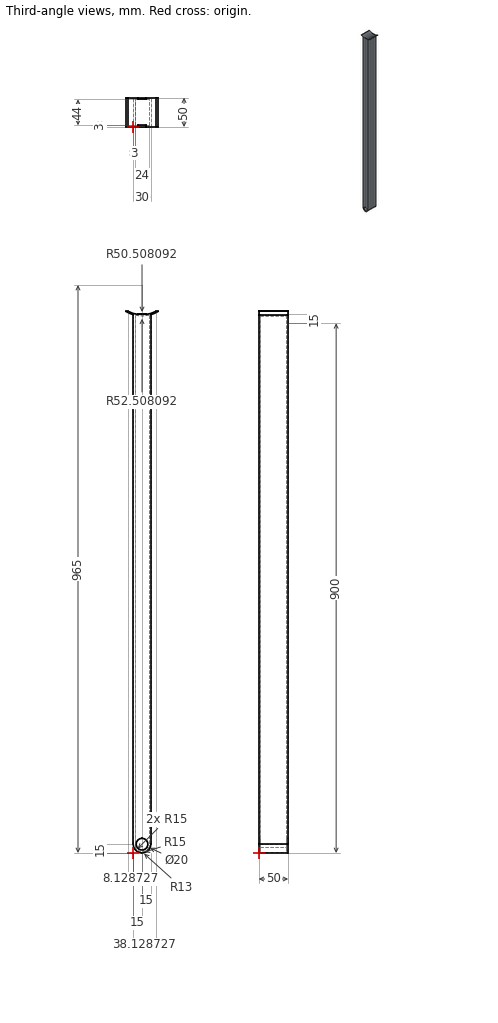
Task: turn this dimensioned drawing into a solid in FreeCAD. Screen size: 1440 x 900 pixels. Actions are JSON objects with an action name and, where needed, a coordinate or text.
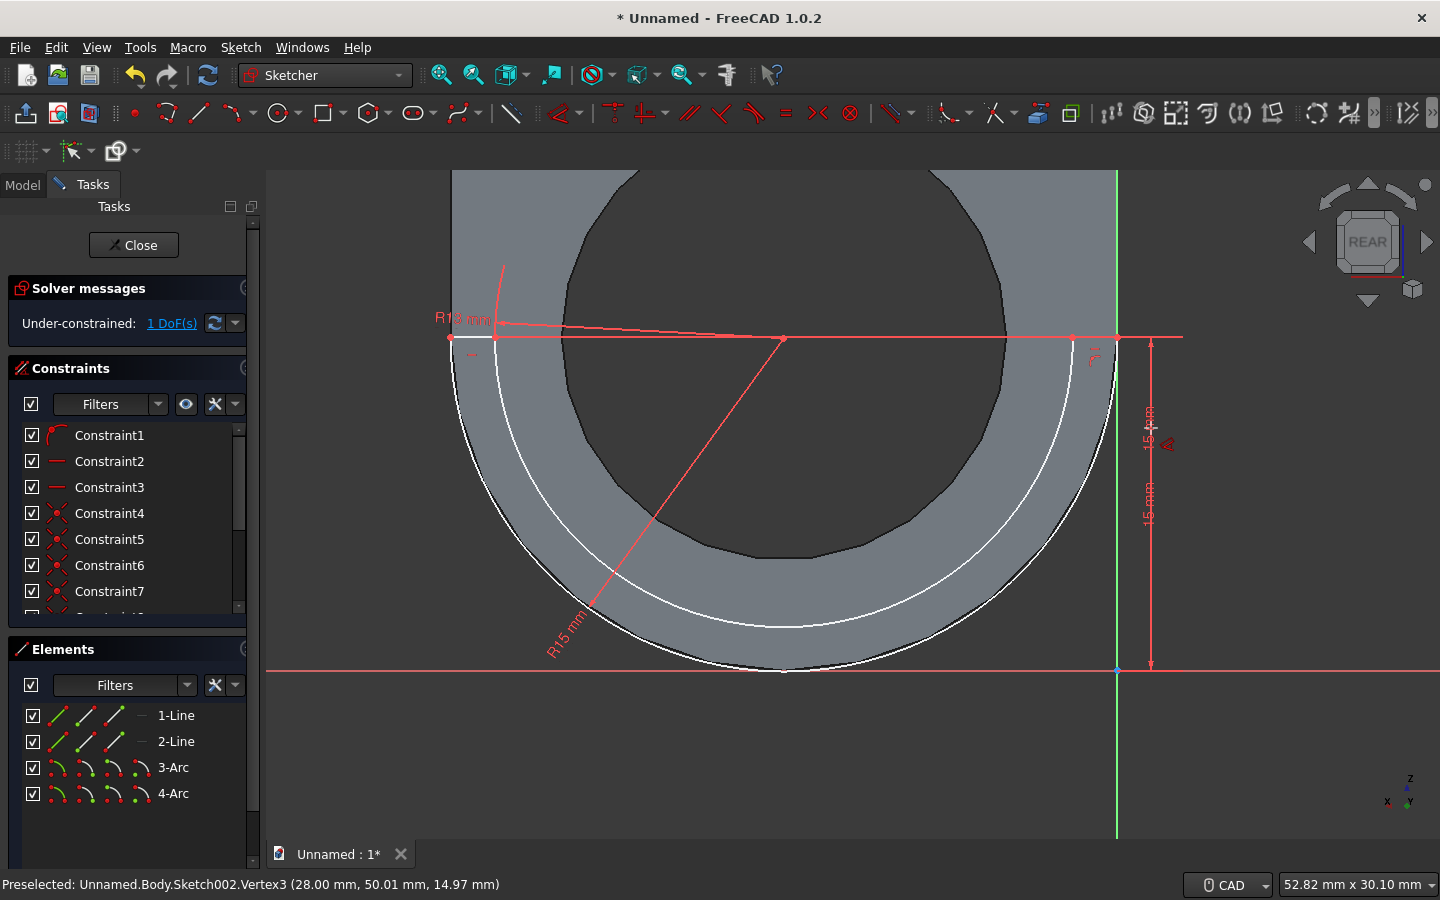
{"action": "left_click", "coordinate": [784, 338]}
{"action": "left_click", "coordinate": [1151, 581]}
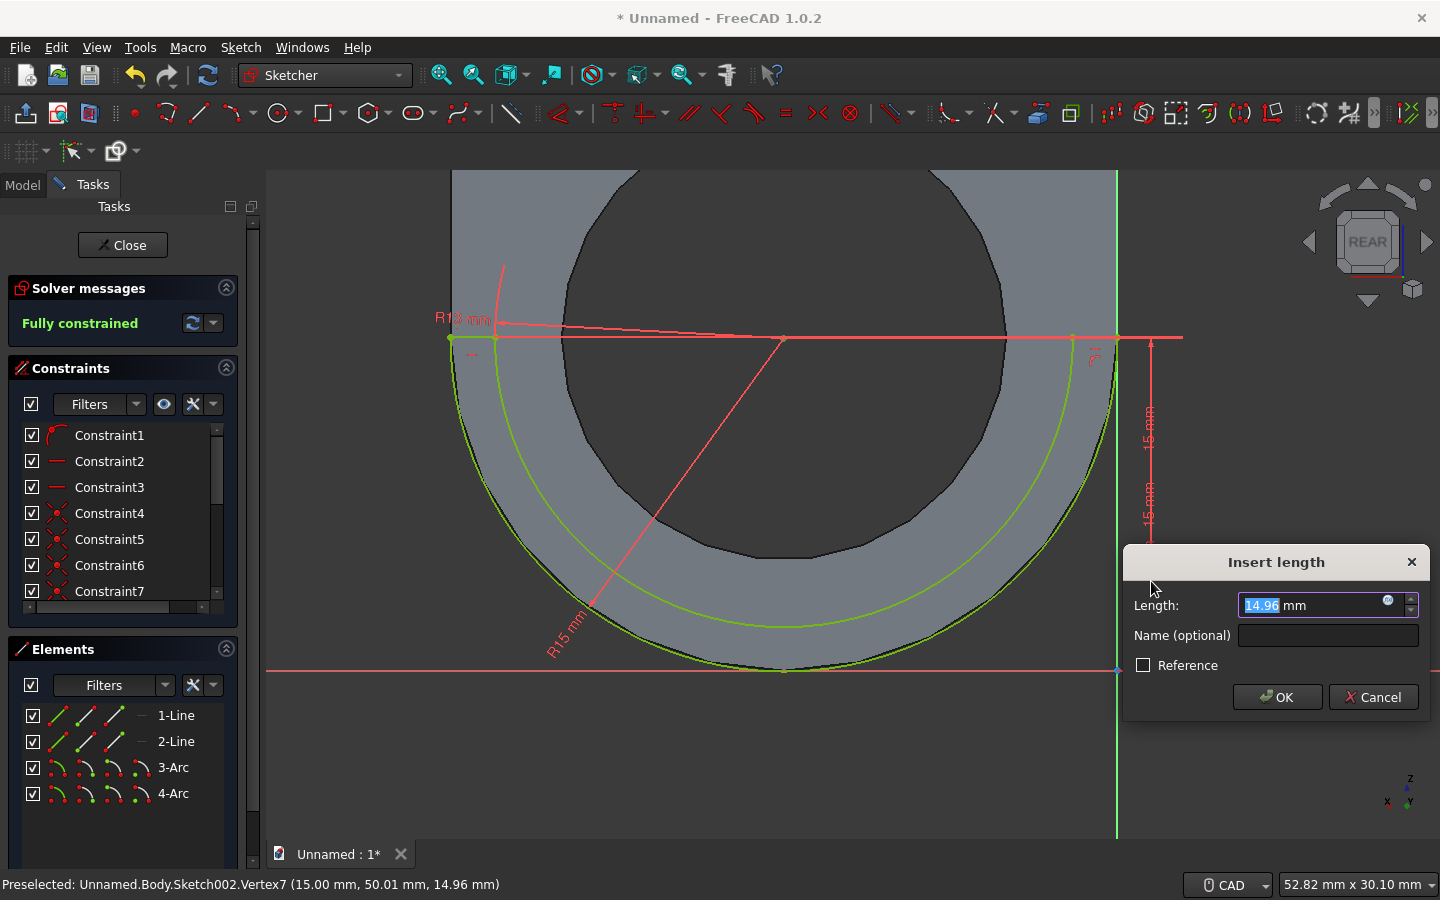
{"action": "type", "text": "15"}
{"action": "key", "text": "Return"}
{"action": "key", "text": "Escape"}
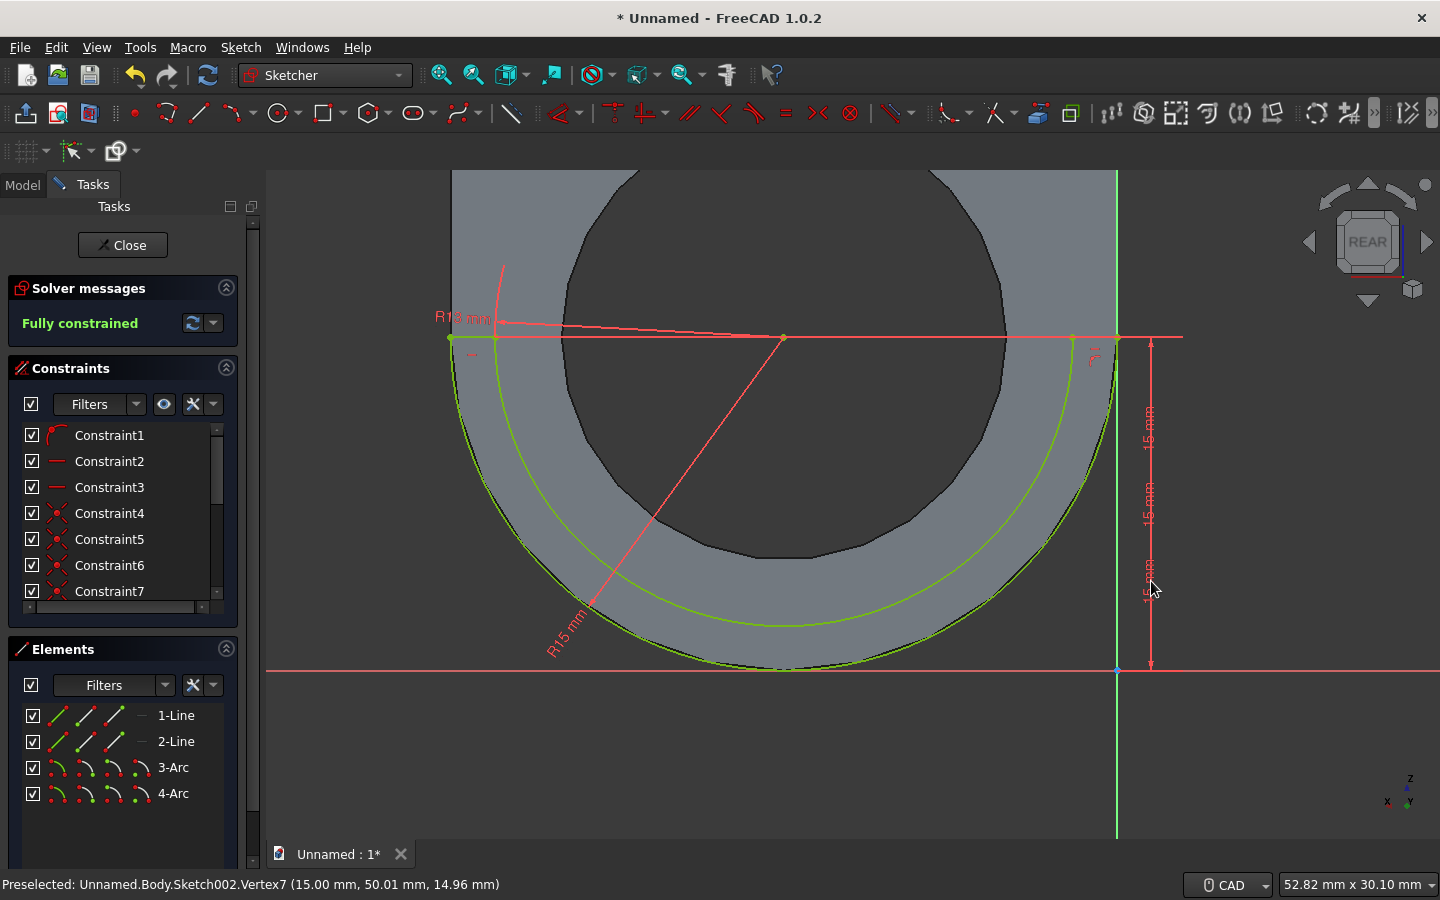
{"action": "left_click", "coordinate": [123, 245]}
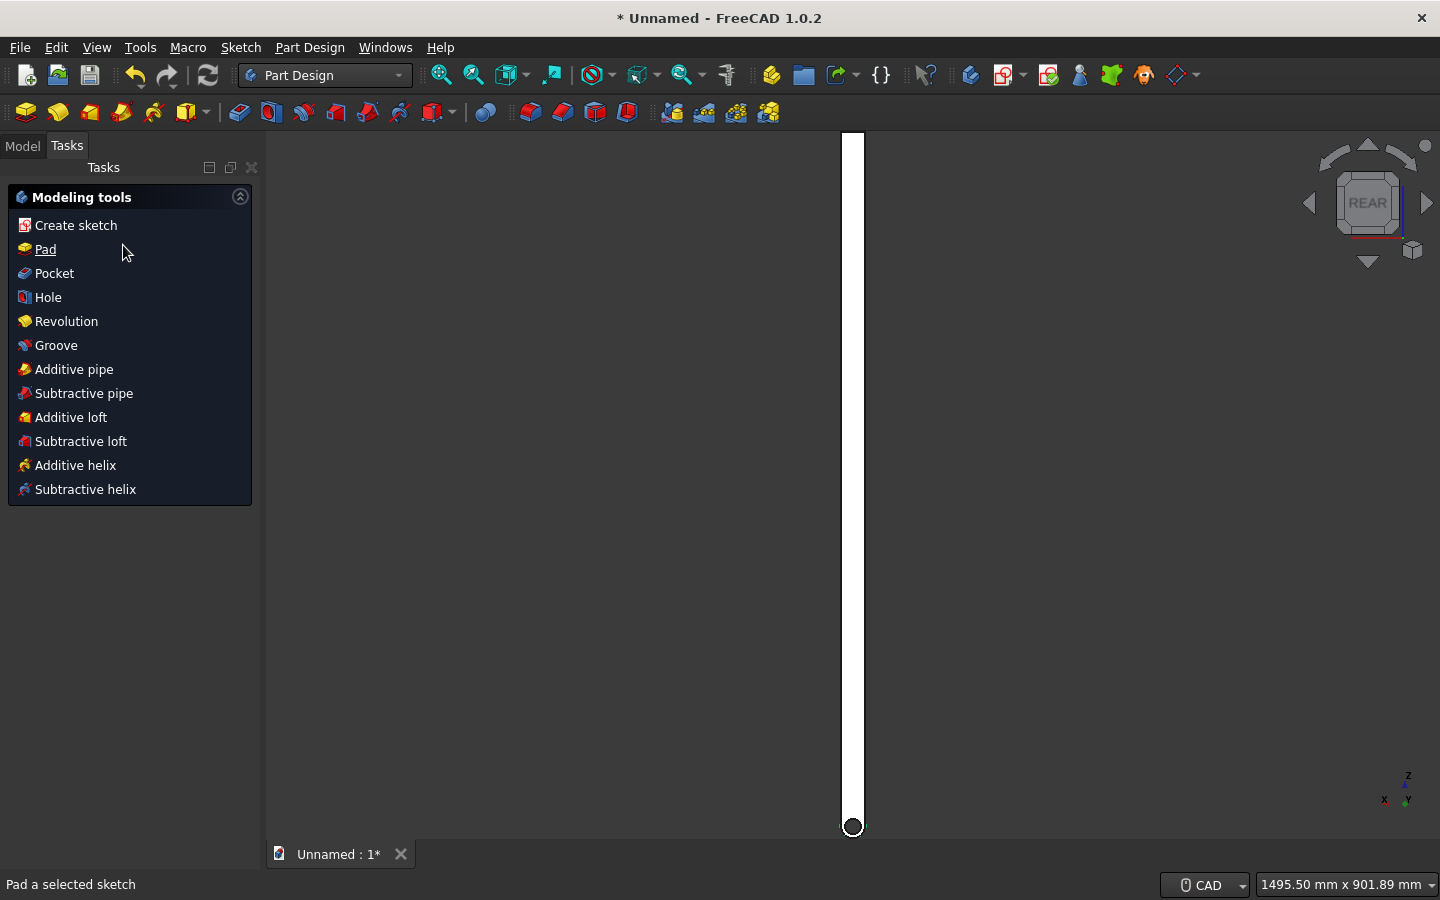
{"action": "left_click", "coordinate": [26, 112]}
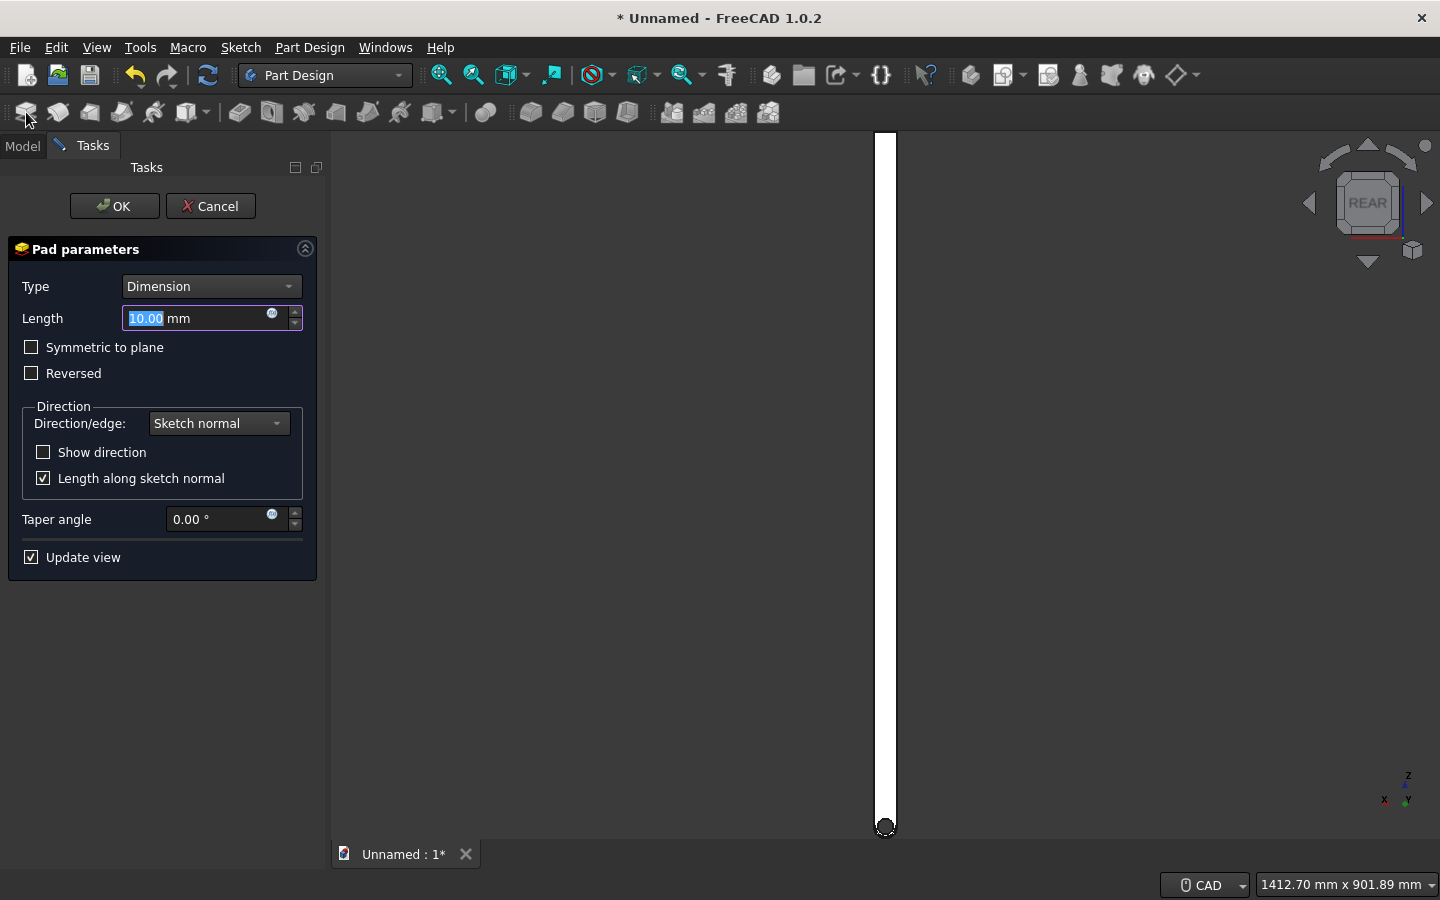
{"action": "type", "text": "50"}
{"action": "key", "text": "Tab"}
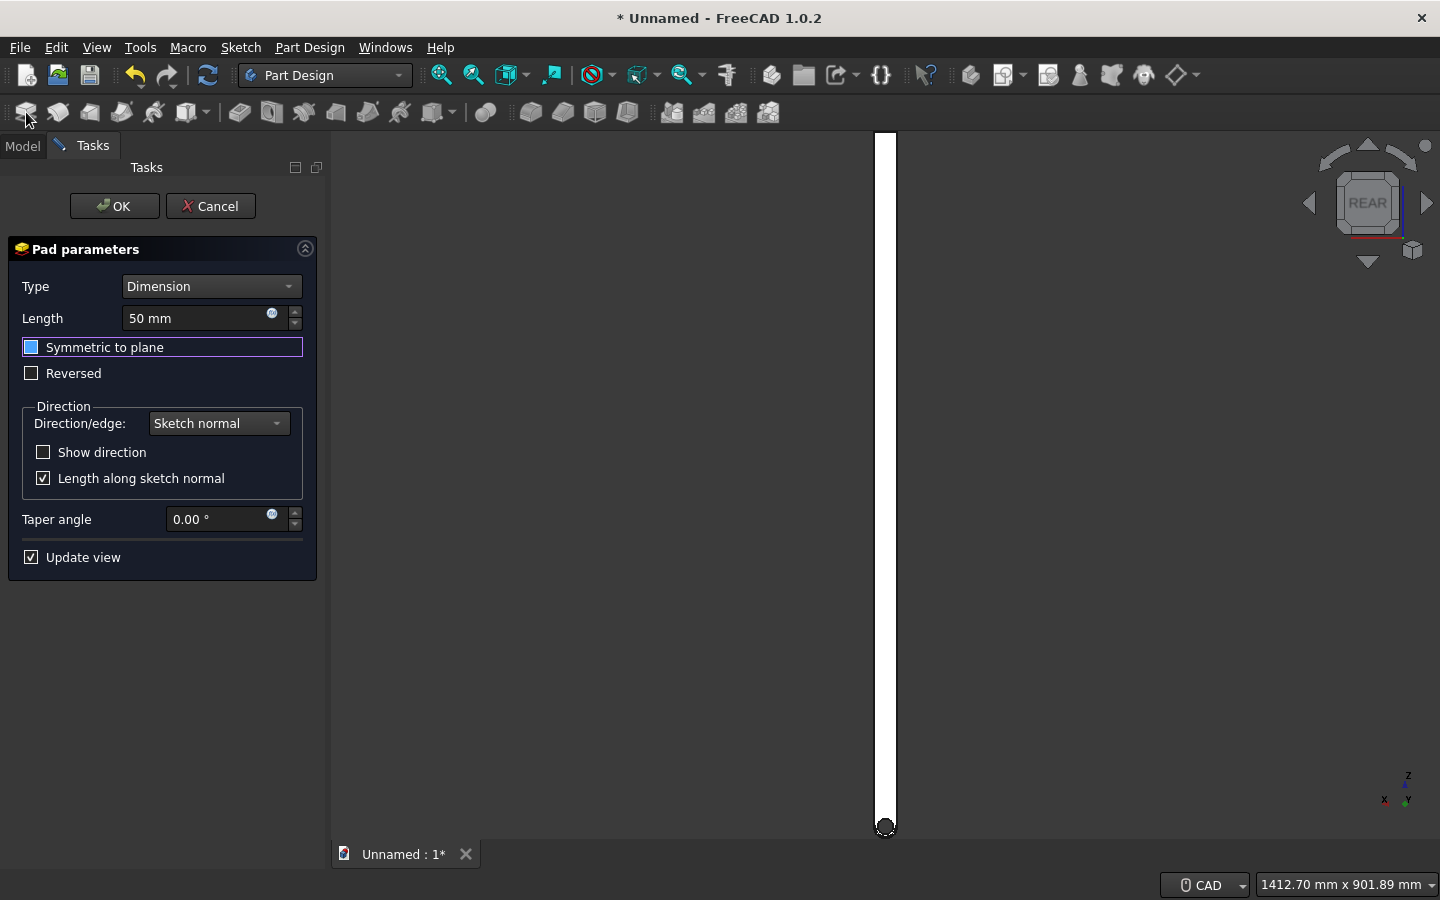
{"action": "left_click", "coordinate": [30, 373]}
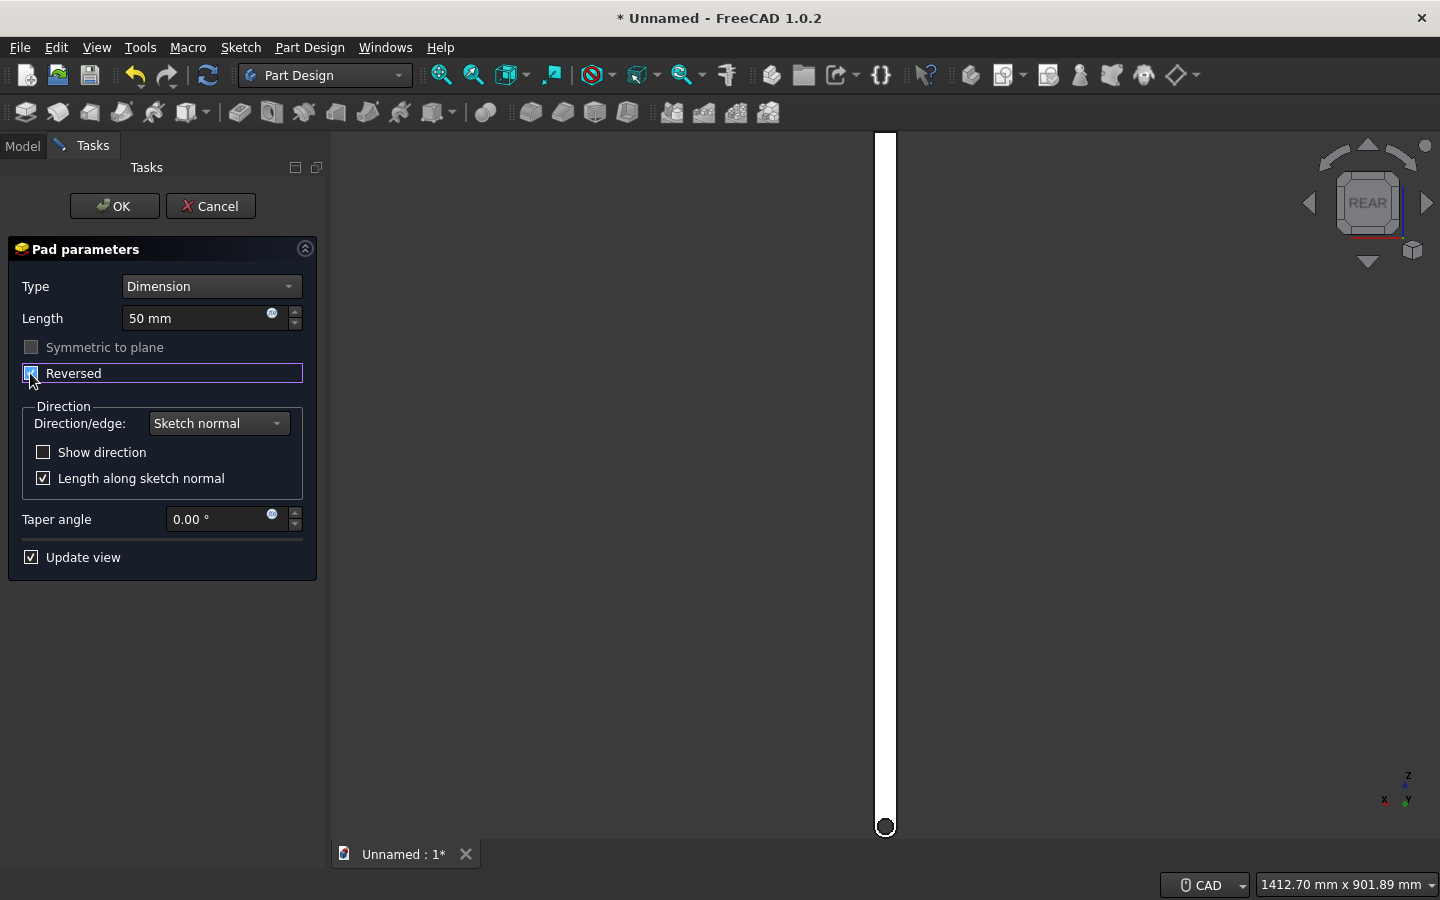
{"action": "left_click", "coordinate": [115, 206]}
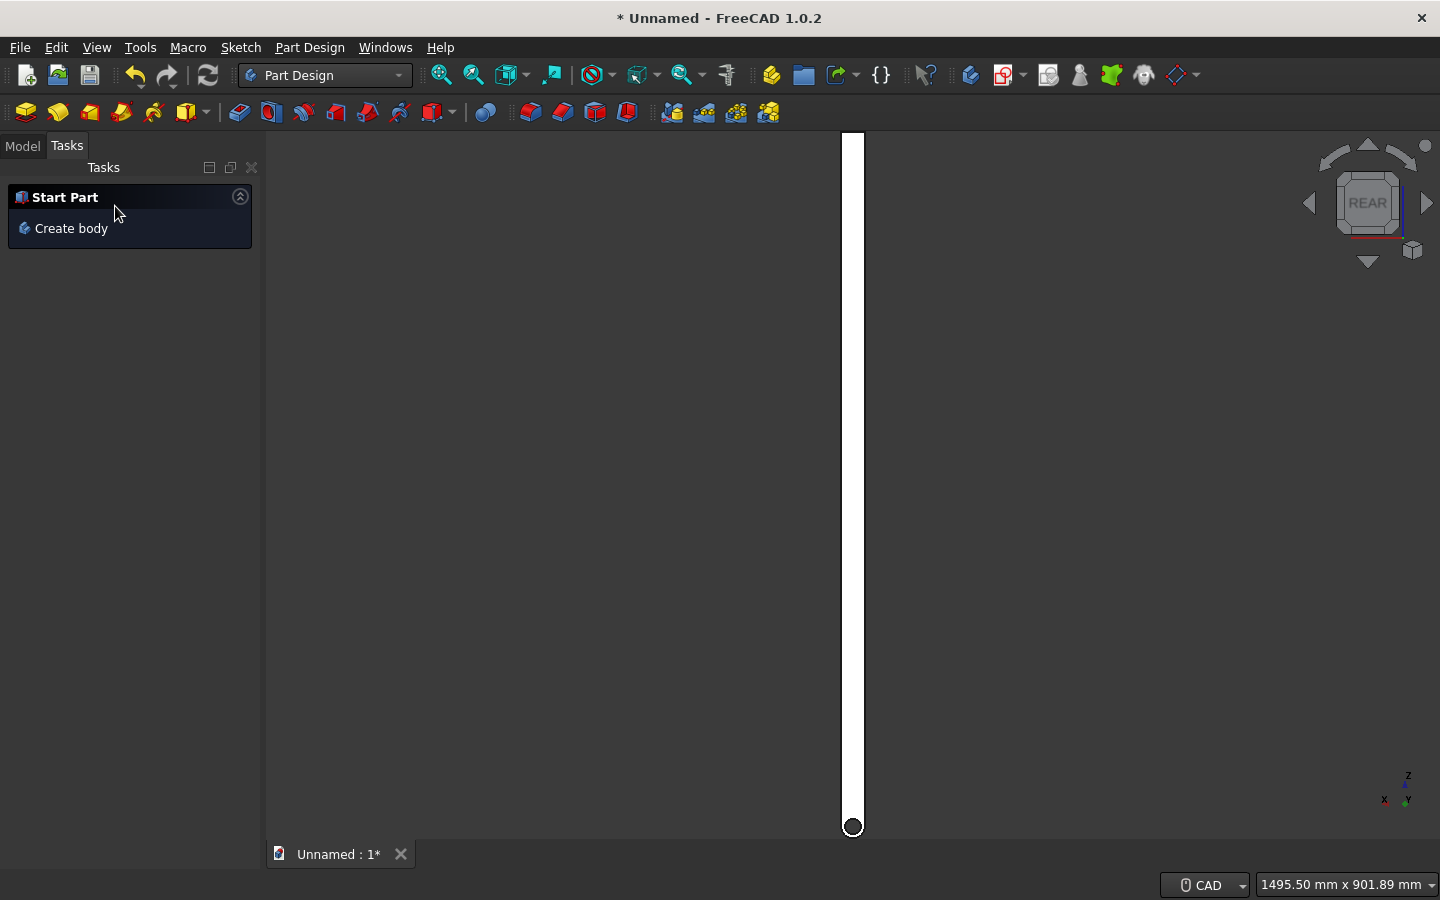
{"action": "key", "text": "0"}